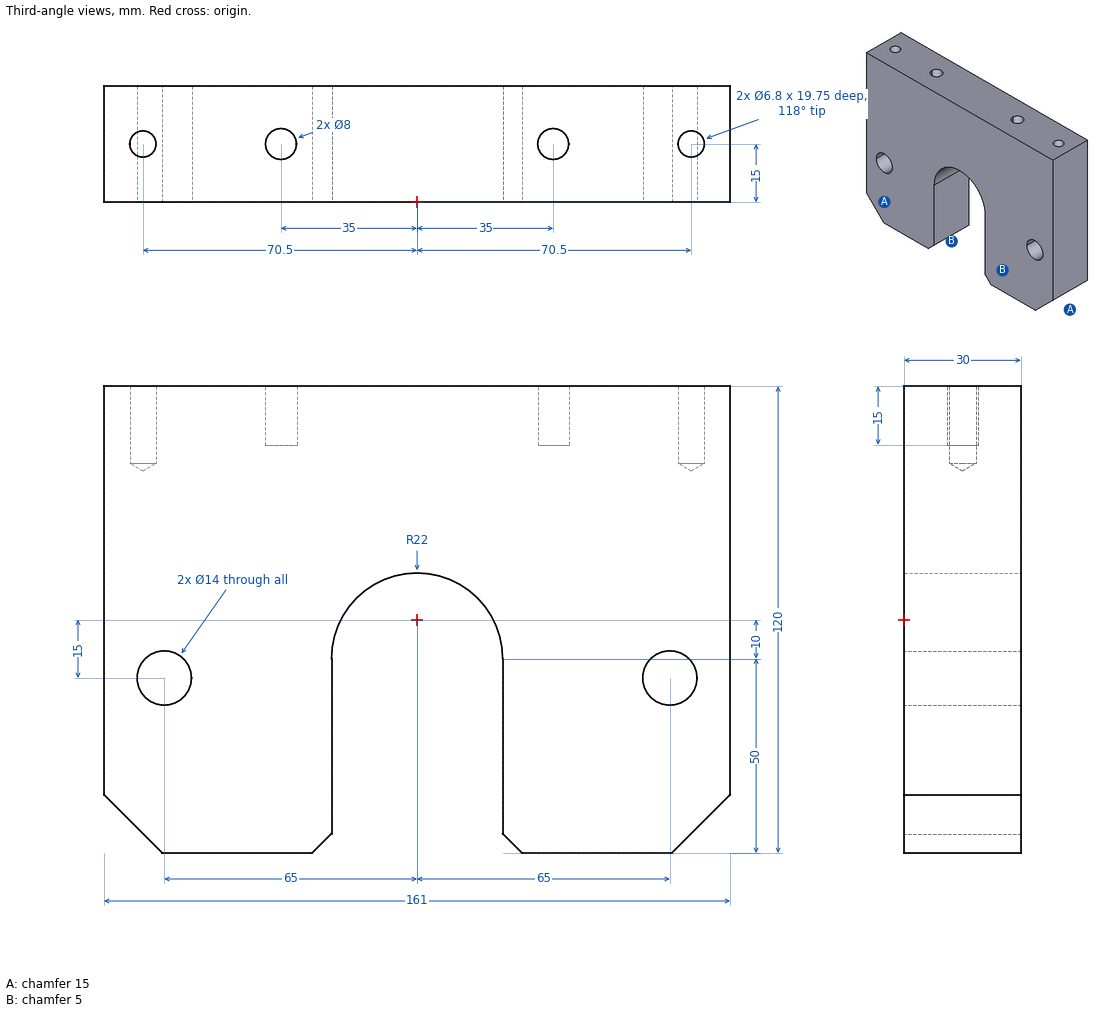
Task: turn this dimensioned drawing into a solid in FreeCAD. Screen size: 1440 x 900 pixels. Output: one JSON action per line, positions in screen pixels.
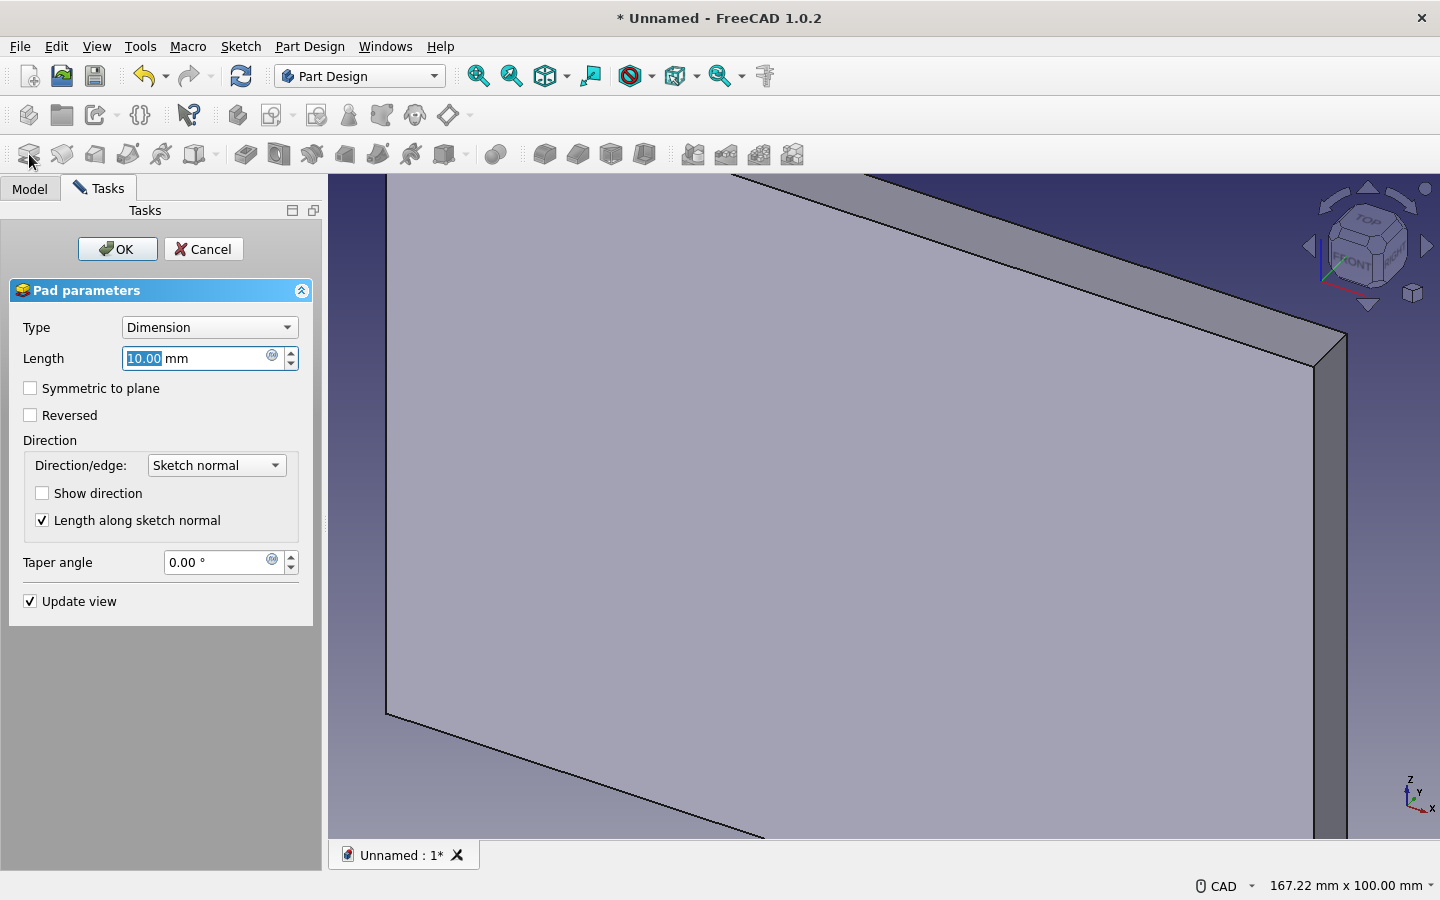
{"action": "type", "text": "30"}
{"action": "key", "text": "Tab"}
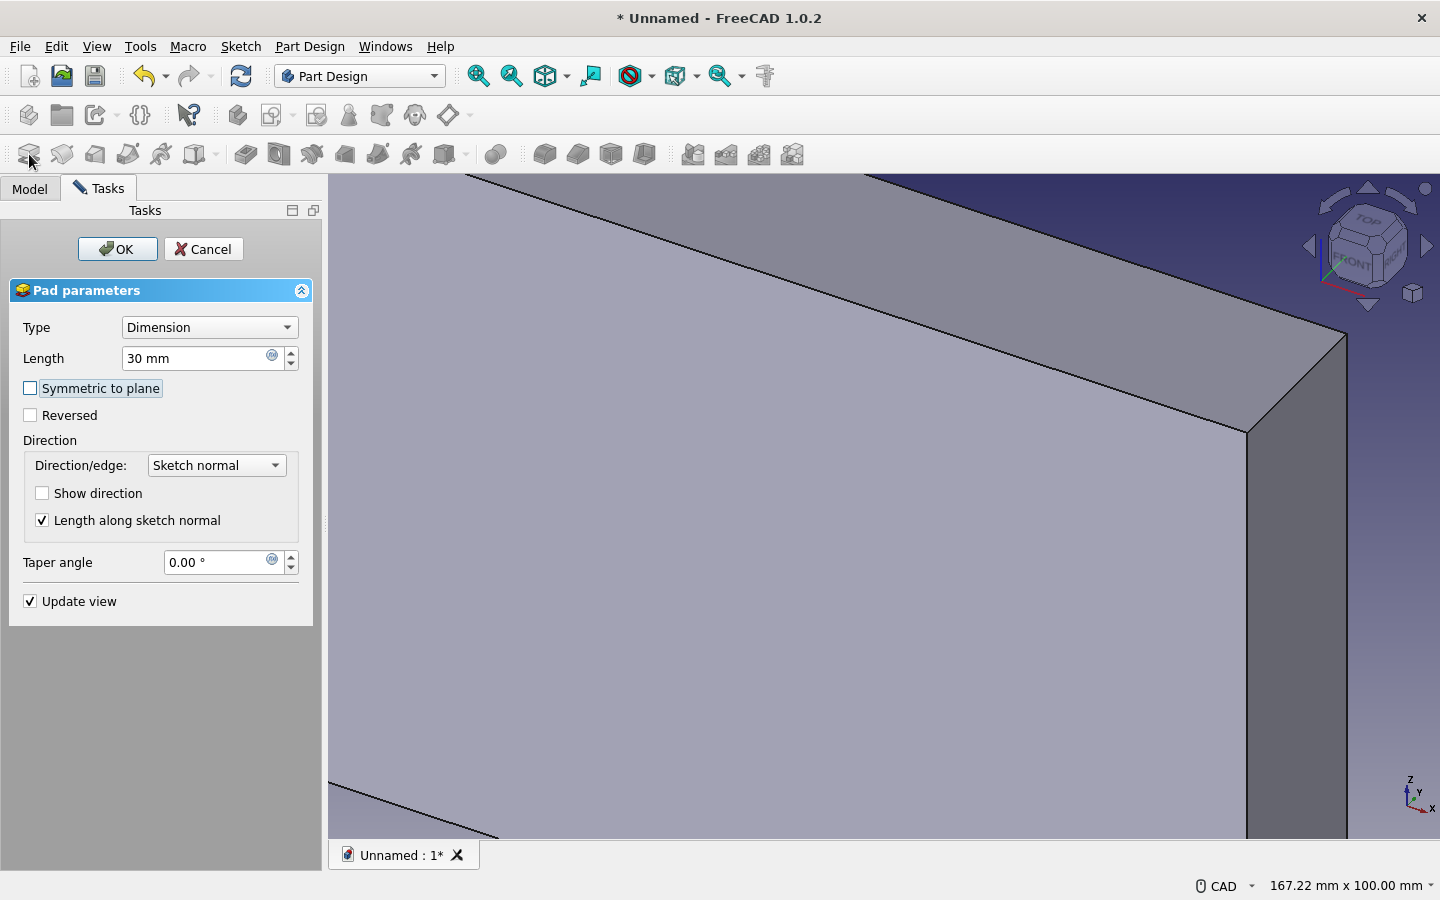
{"action": "left_click", "coordinate": [31, 415]}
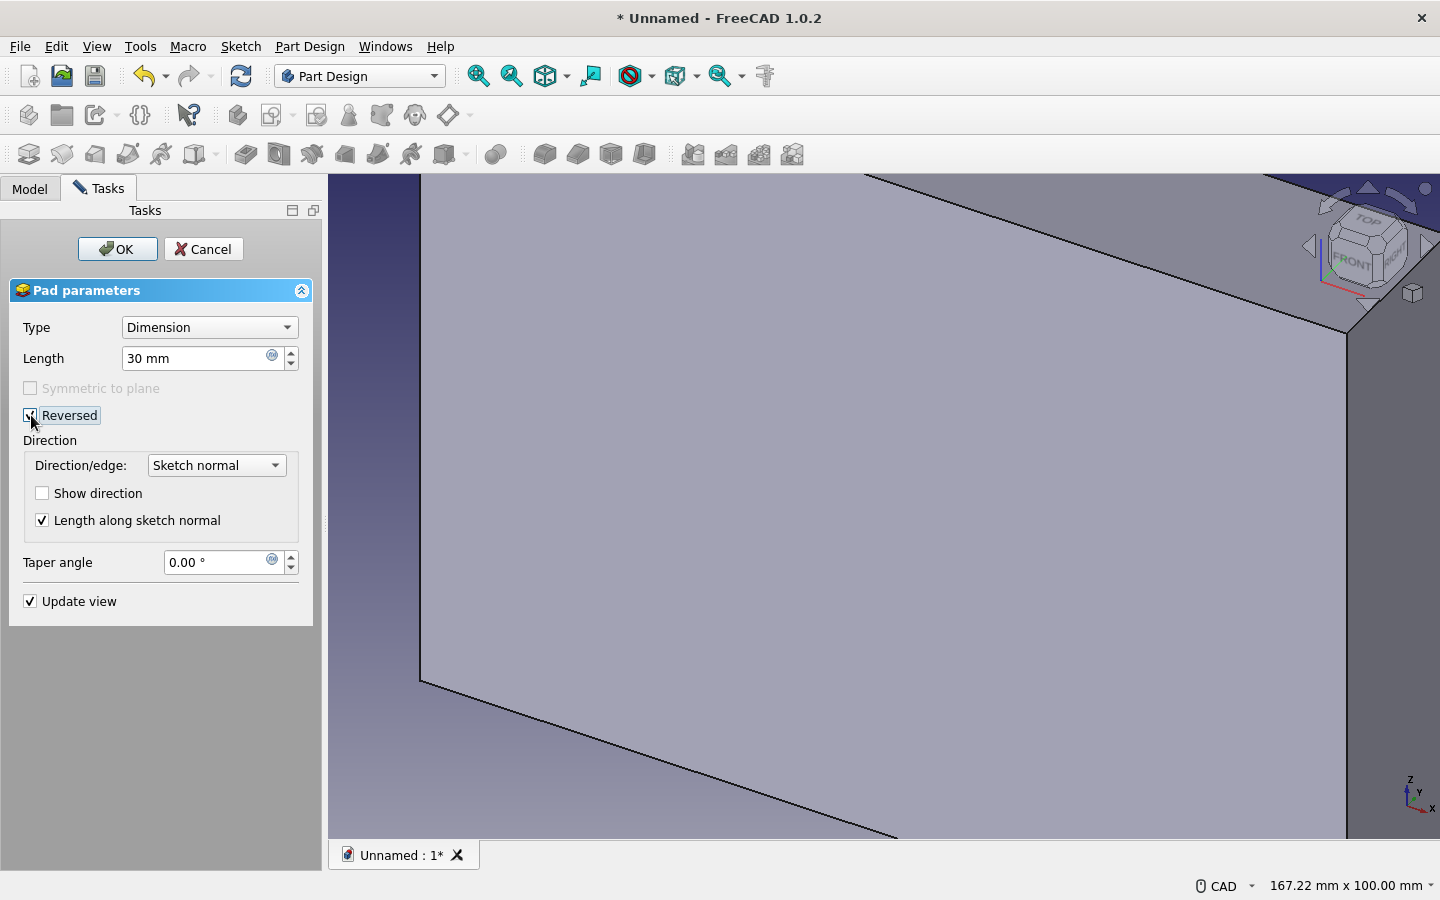
{"action": "left_click", "coordinate": [118, 249]}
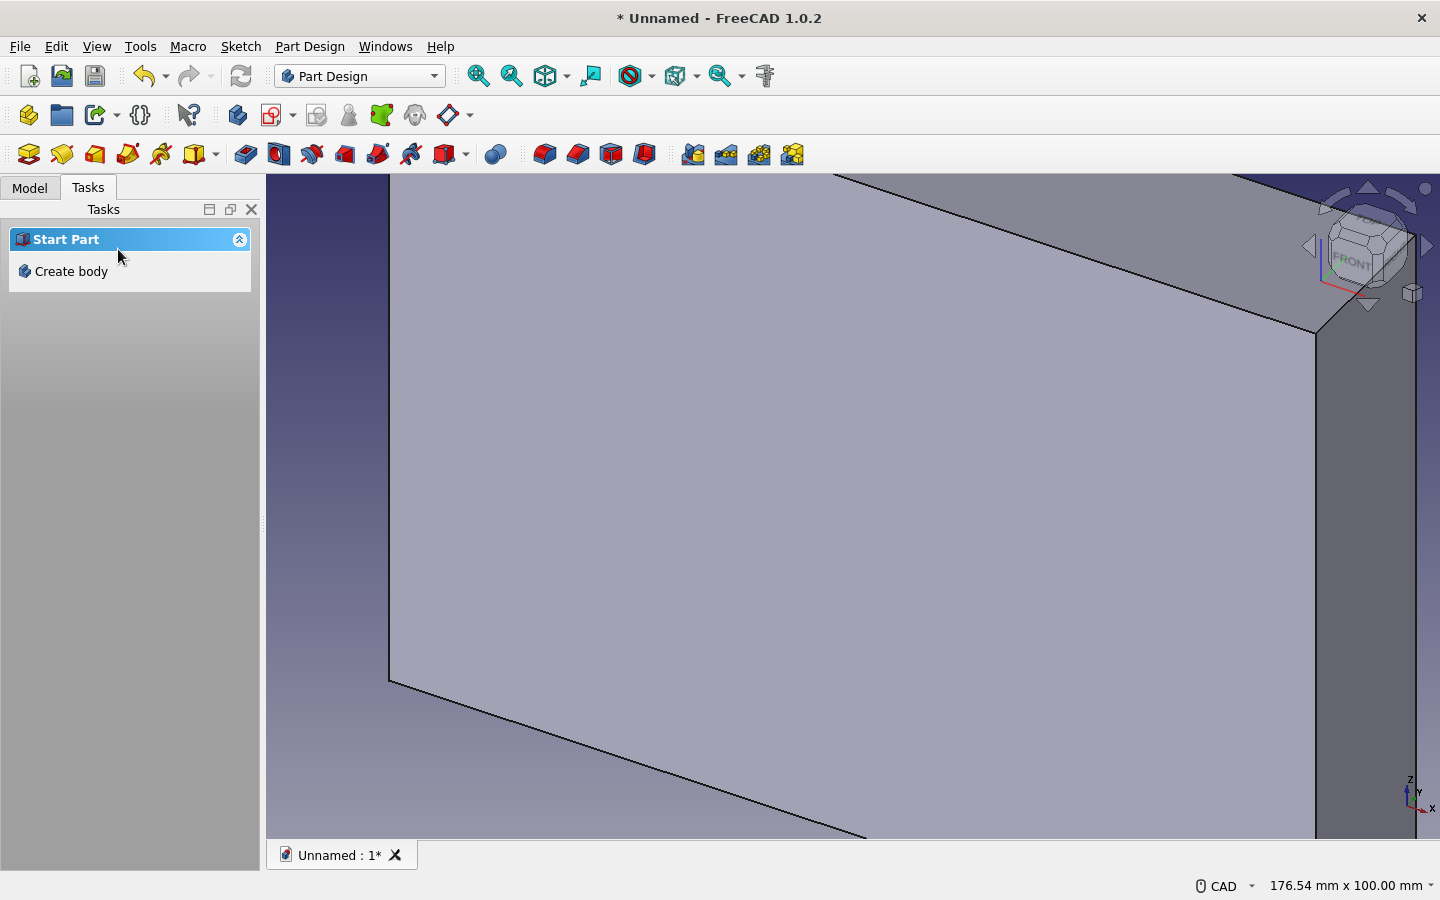
{"action": "key", "text": "v f"}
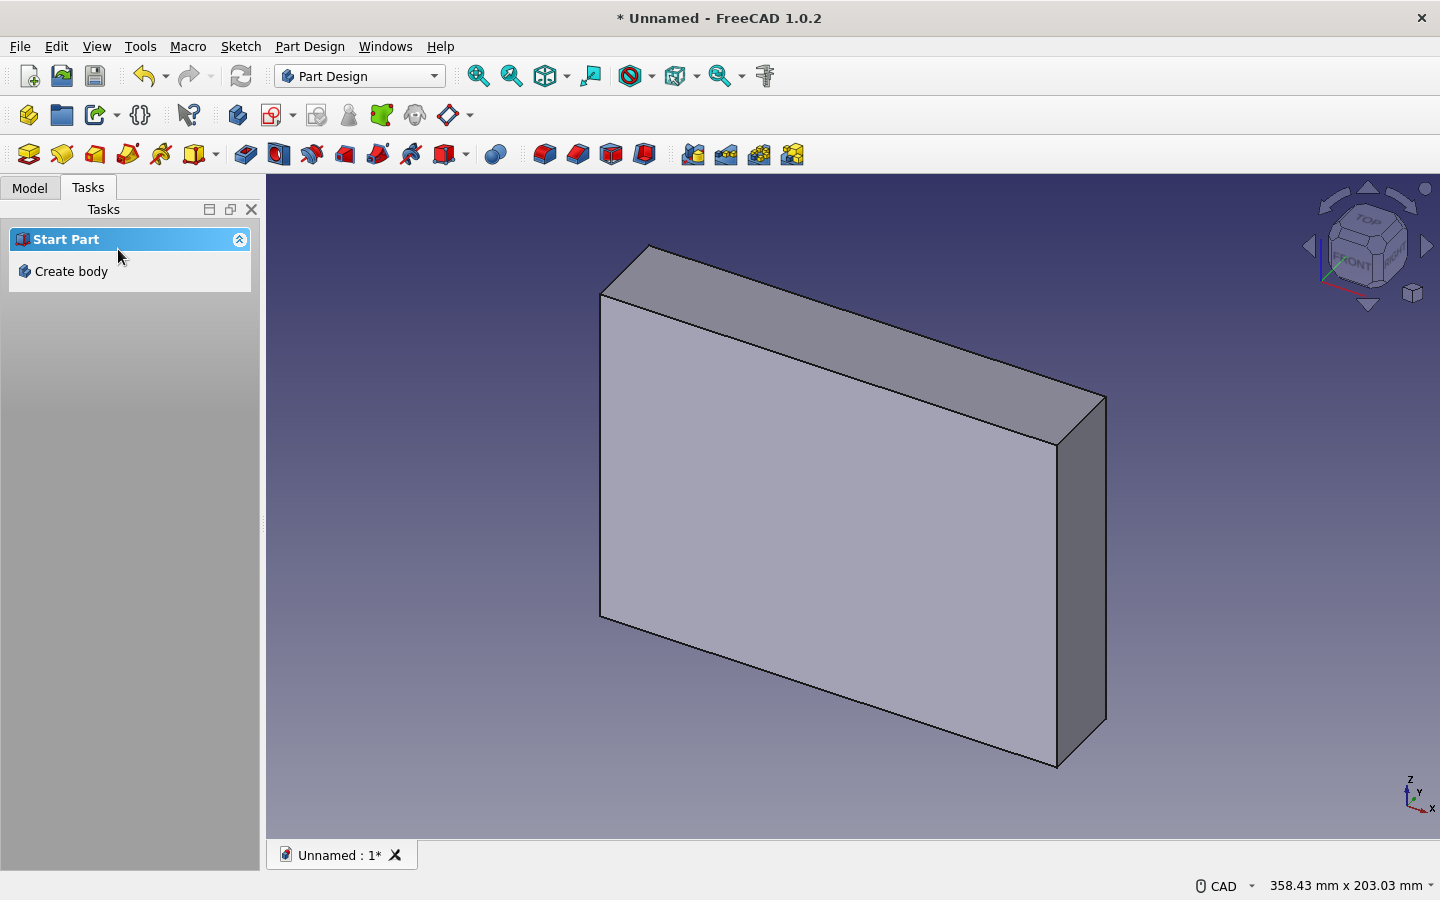
{"action": "key", "text": "4"}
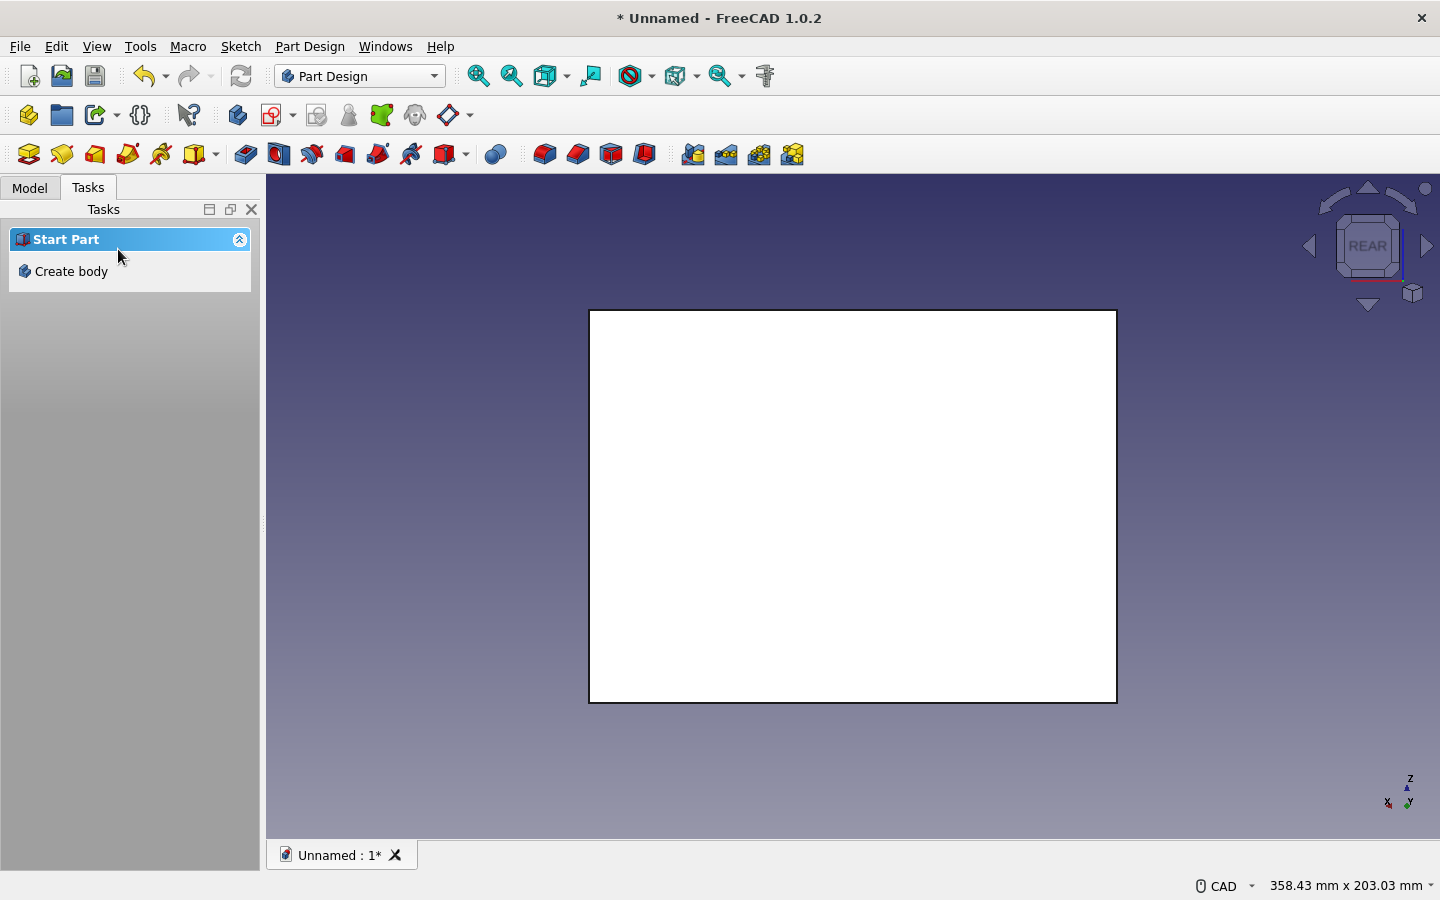
{"action": "left_click", "coordinate": [853, 506]}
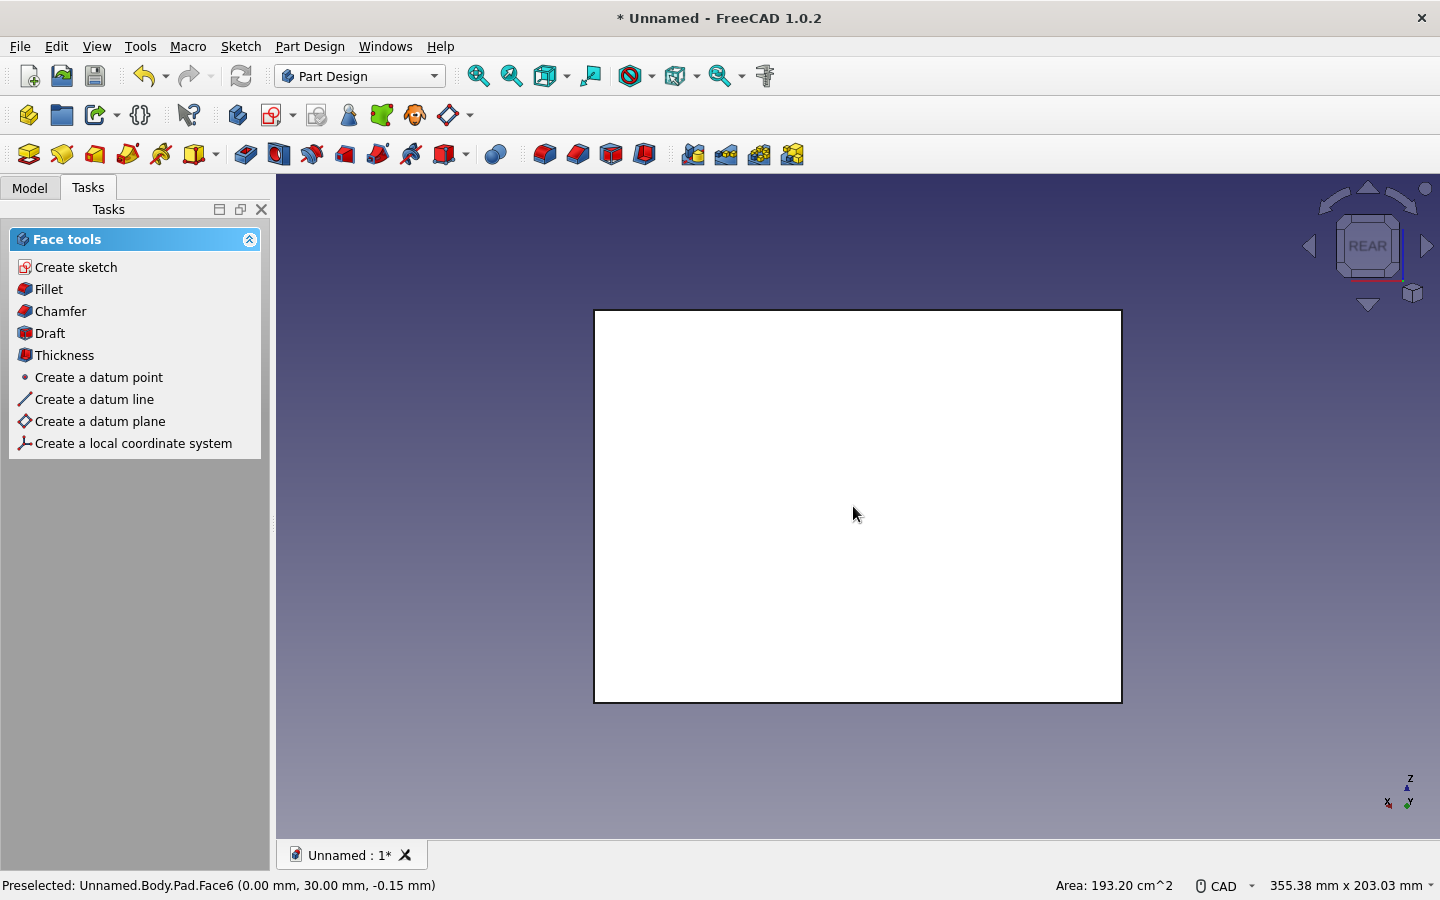
{"action": "left_click", "coordinate": [270, 116]}